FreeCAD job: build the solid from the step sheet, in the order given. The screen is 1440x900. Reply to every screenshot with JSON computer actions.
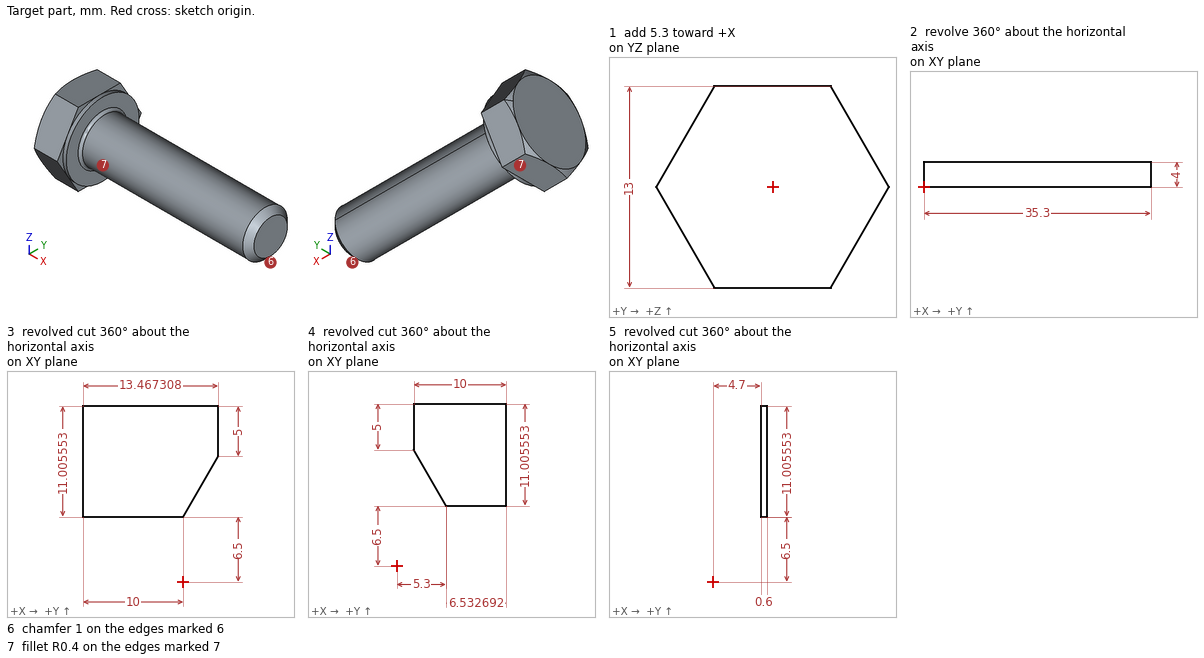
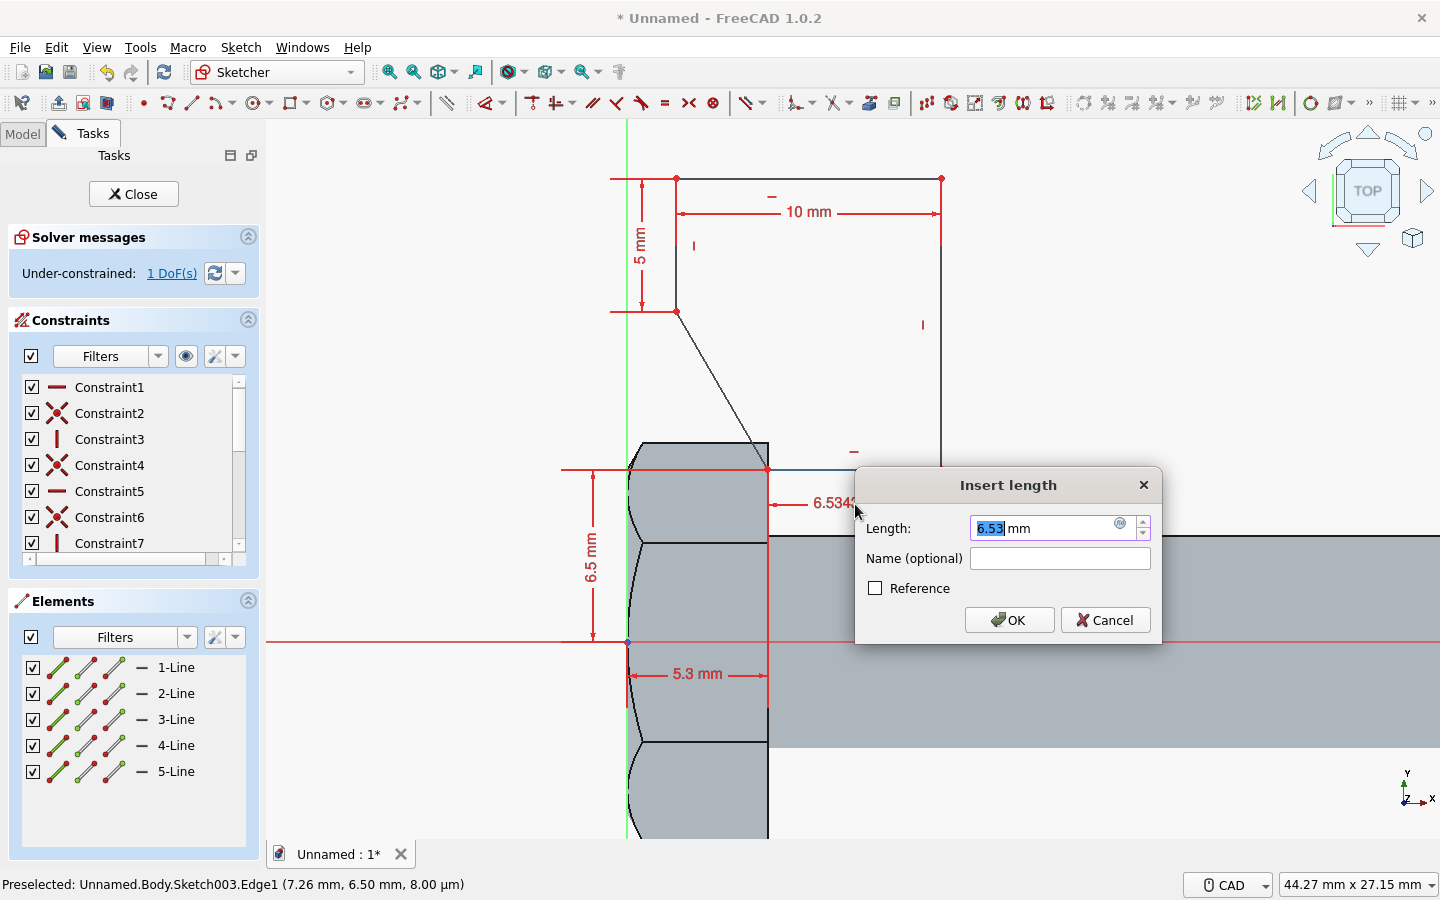
{"action": "type", "text": "6.532692"}
{"action": "key", "text": "Return"}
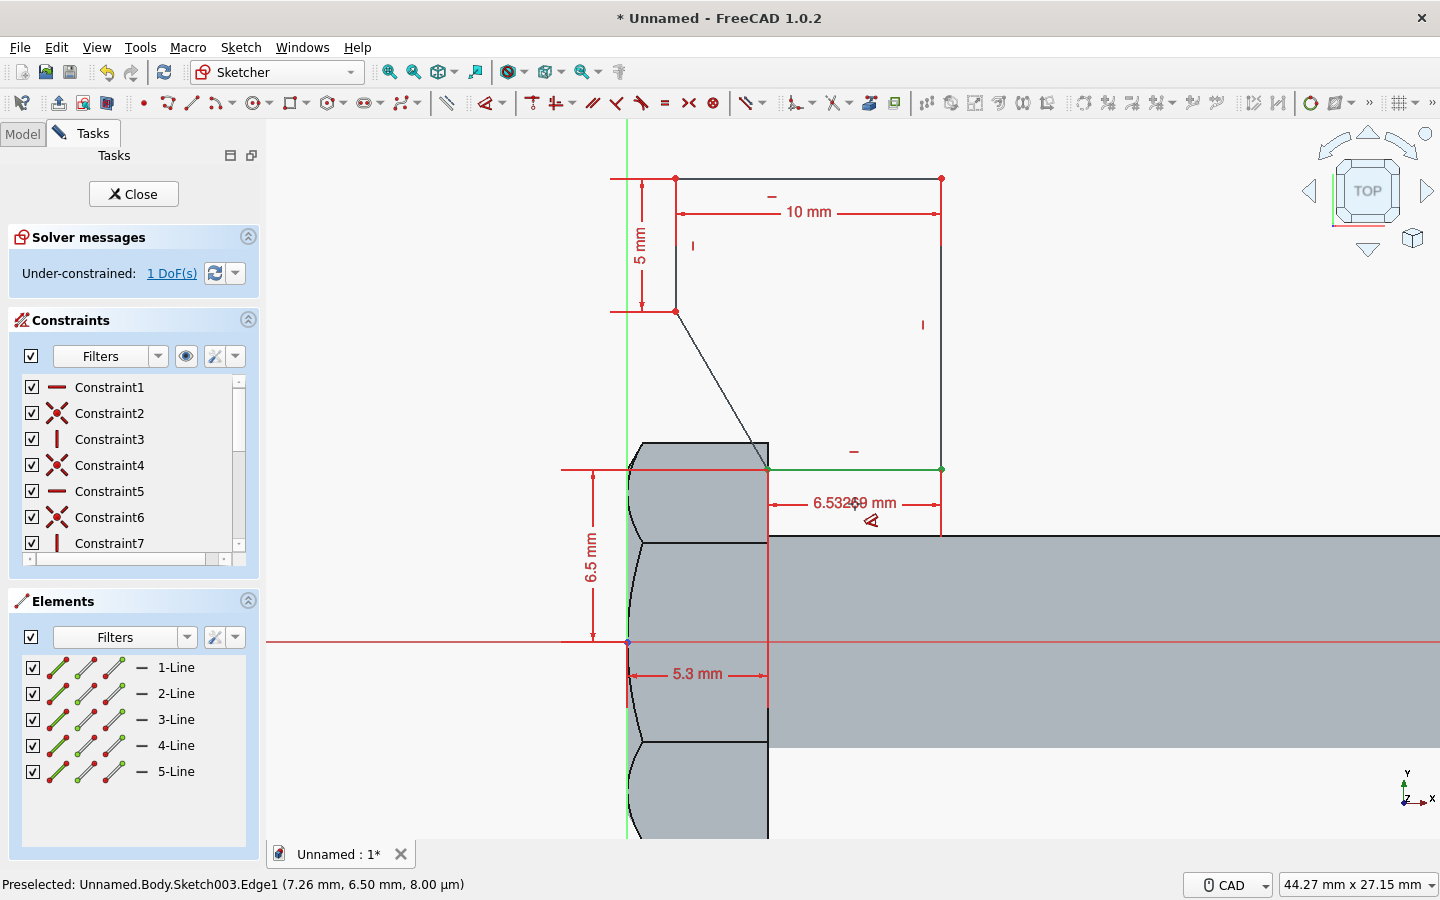
{"action": "left_click", "coordinate": [941, 383]}
{"action": "left_click", "coordinate": [975, 324]}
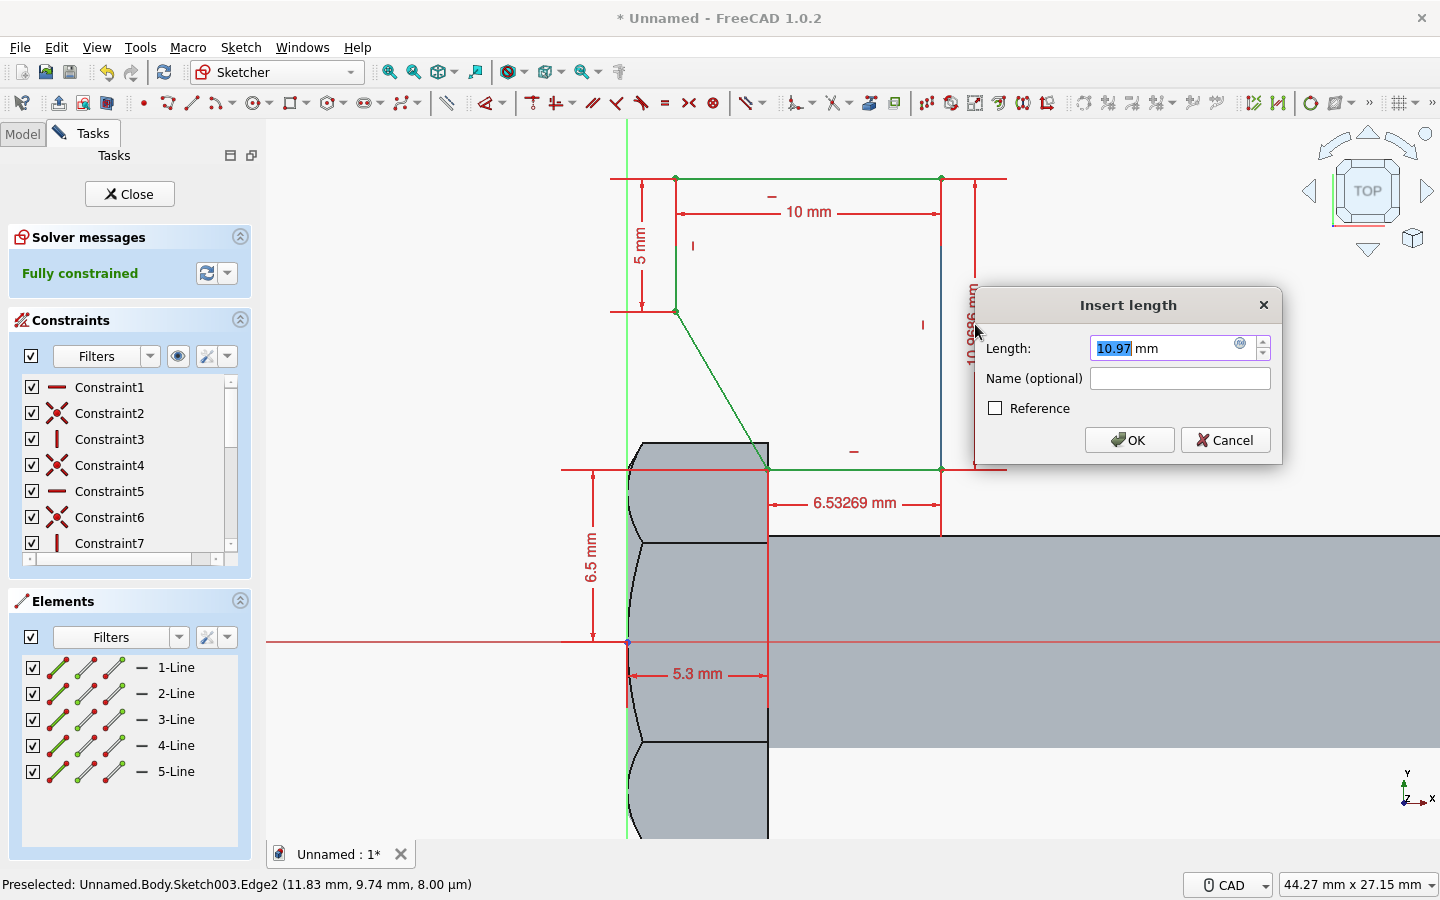
{"action": "type", "text": "11.005553"}
{"action": "key", "text": "Return"}
{"action": "key", "text": "Escape"}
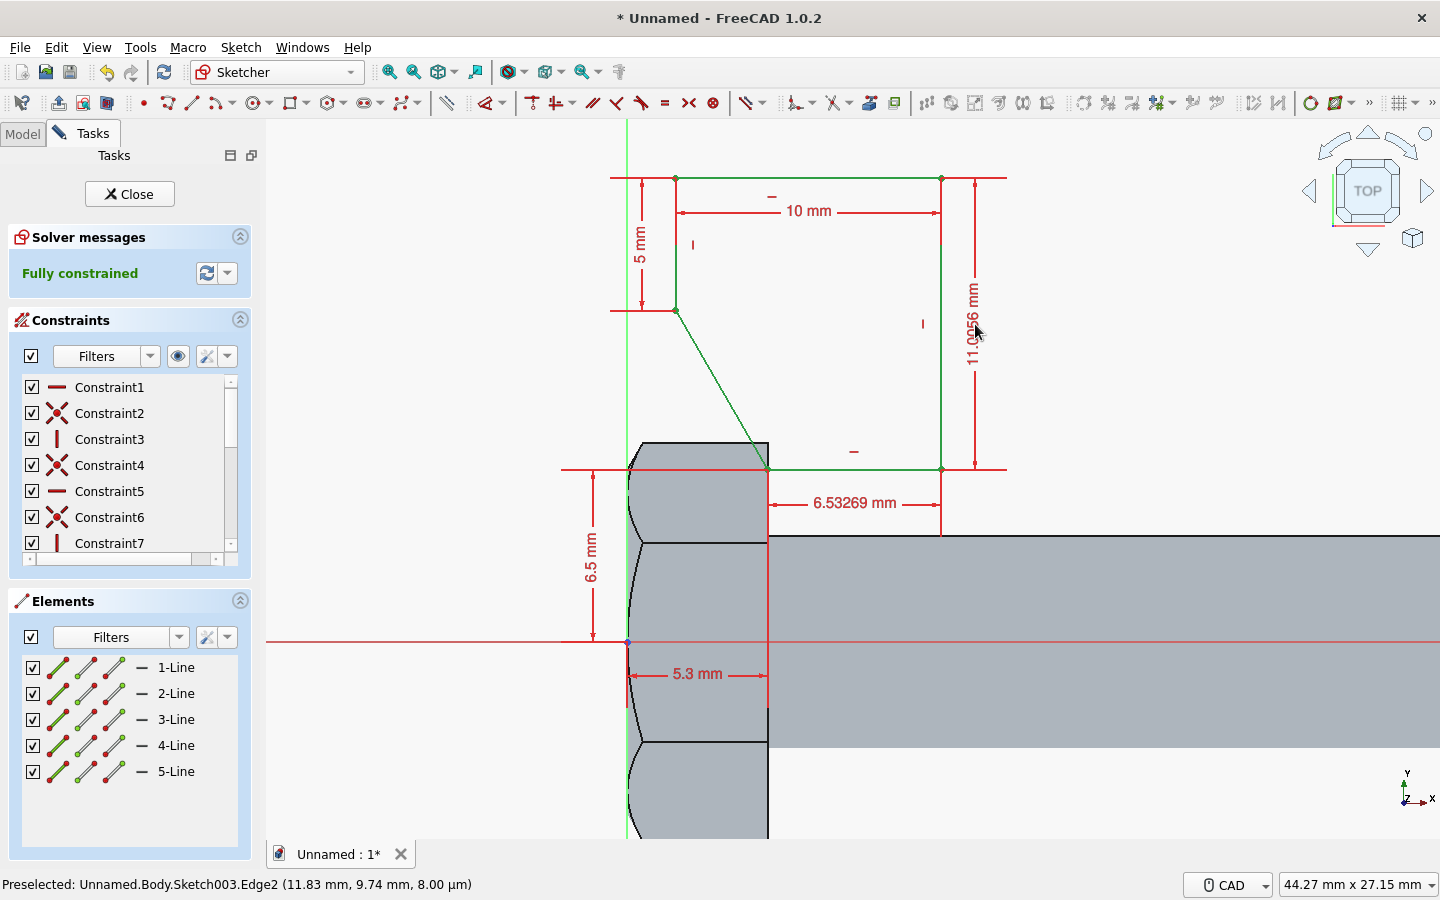
{"action": "left_click", "coordinate": [130, 194]}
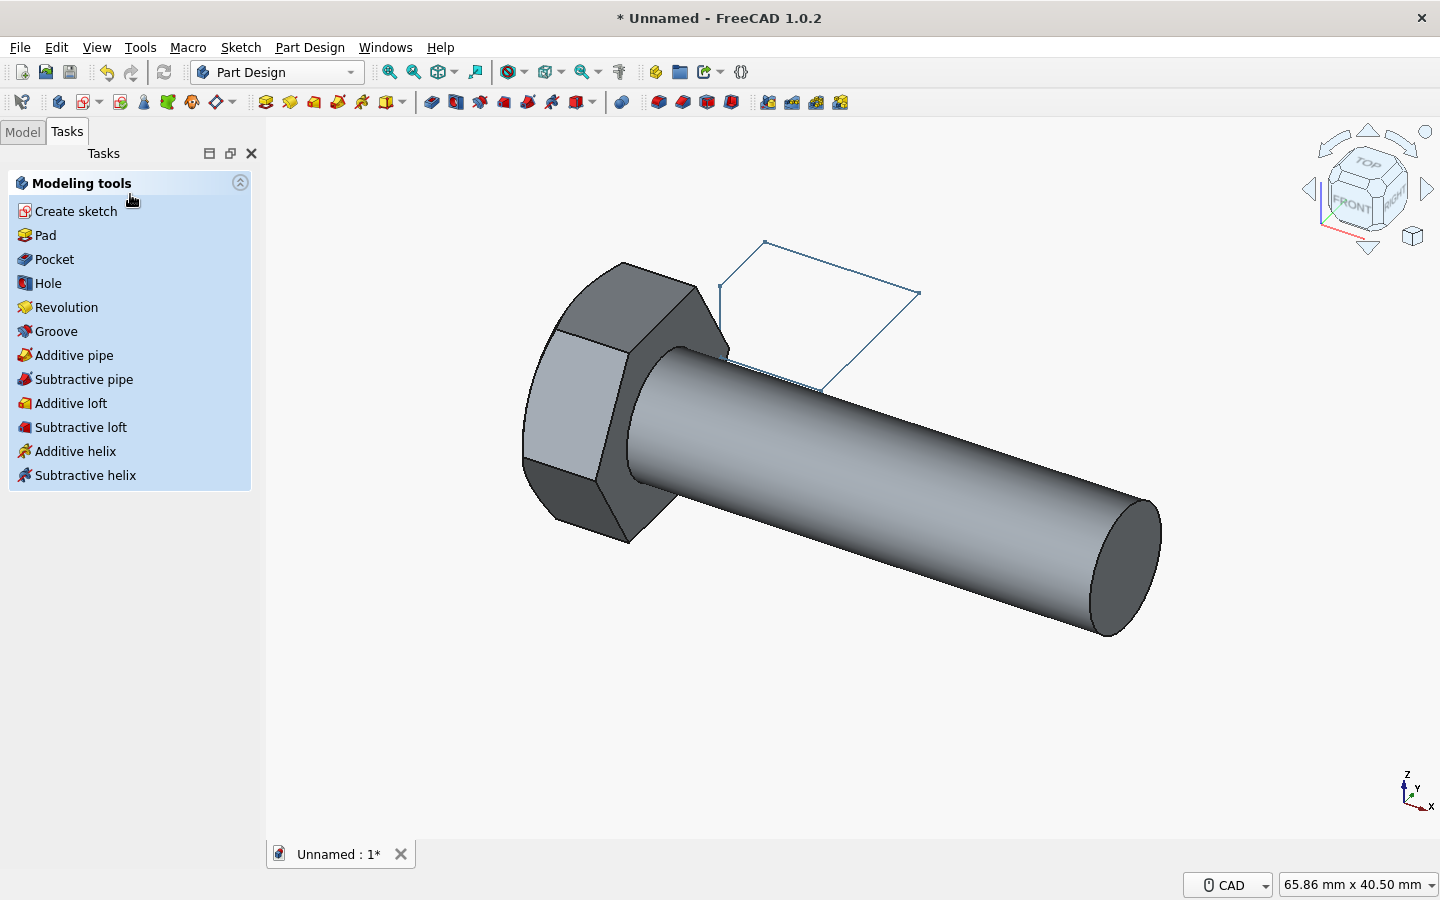
{"action": "left_click", "coordinate": [480, 102]}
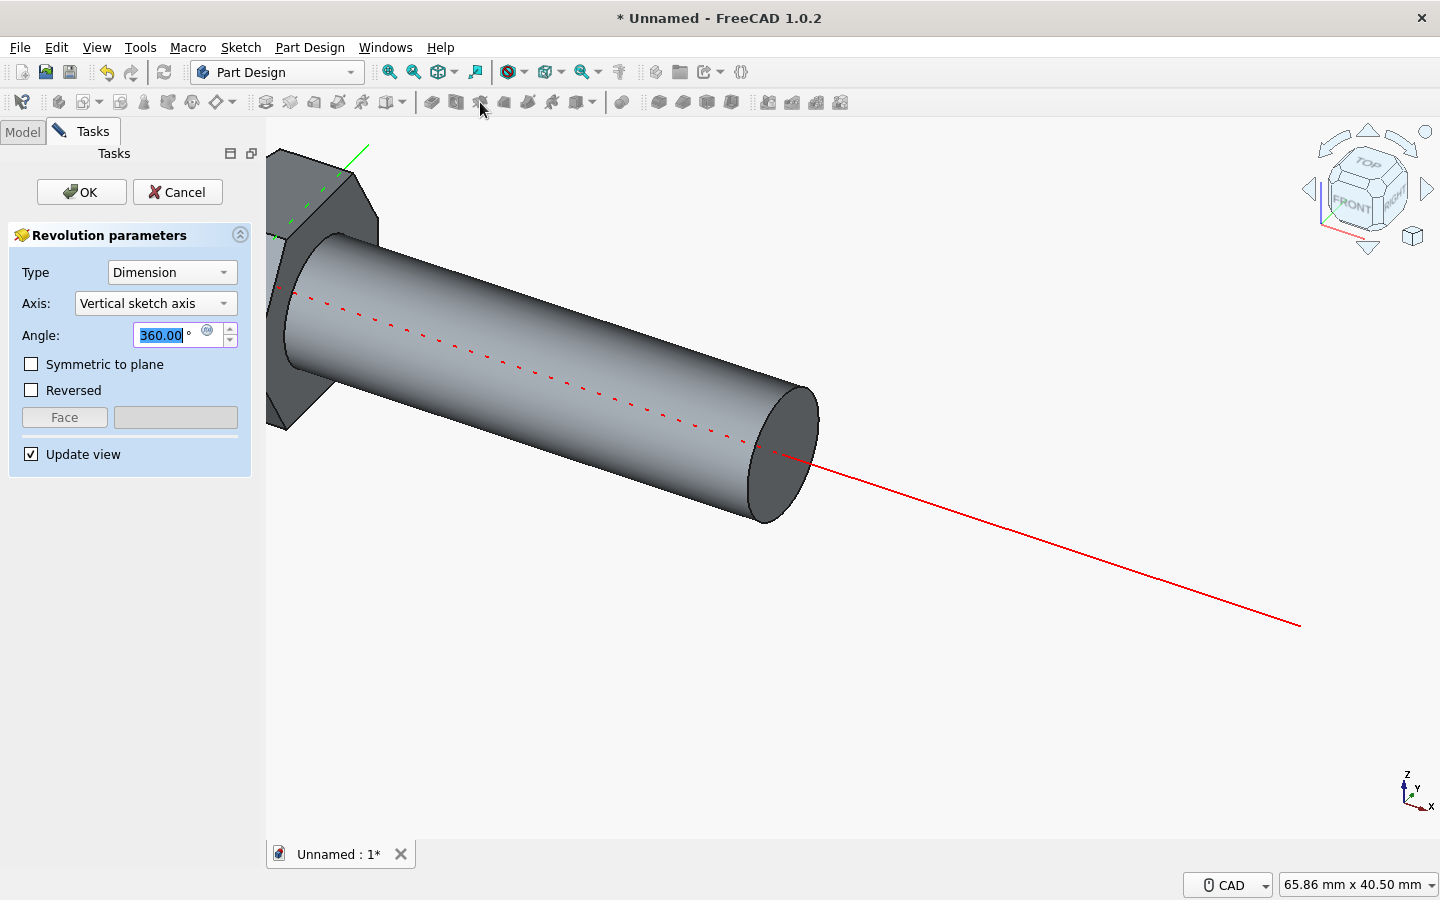
{"action": "left_click", "coordinate": [156, 304]}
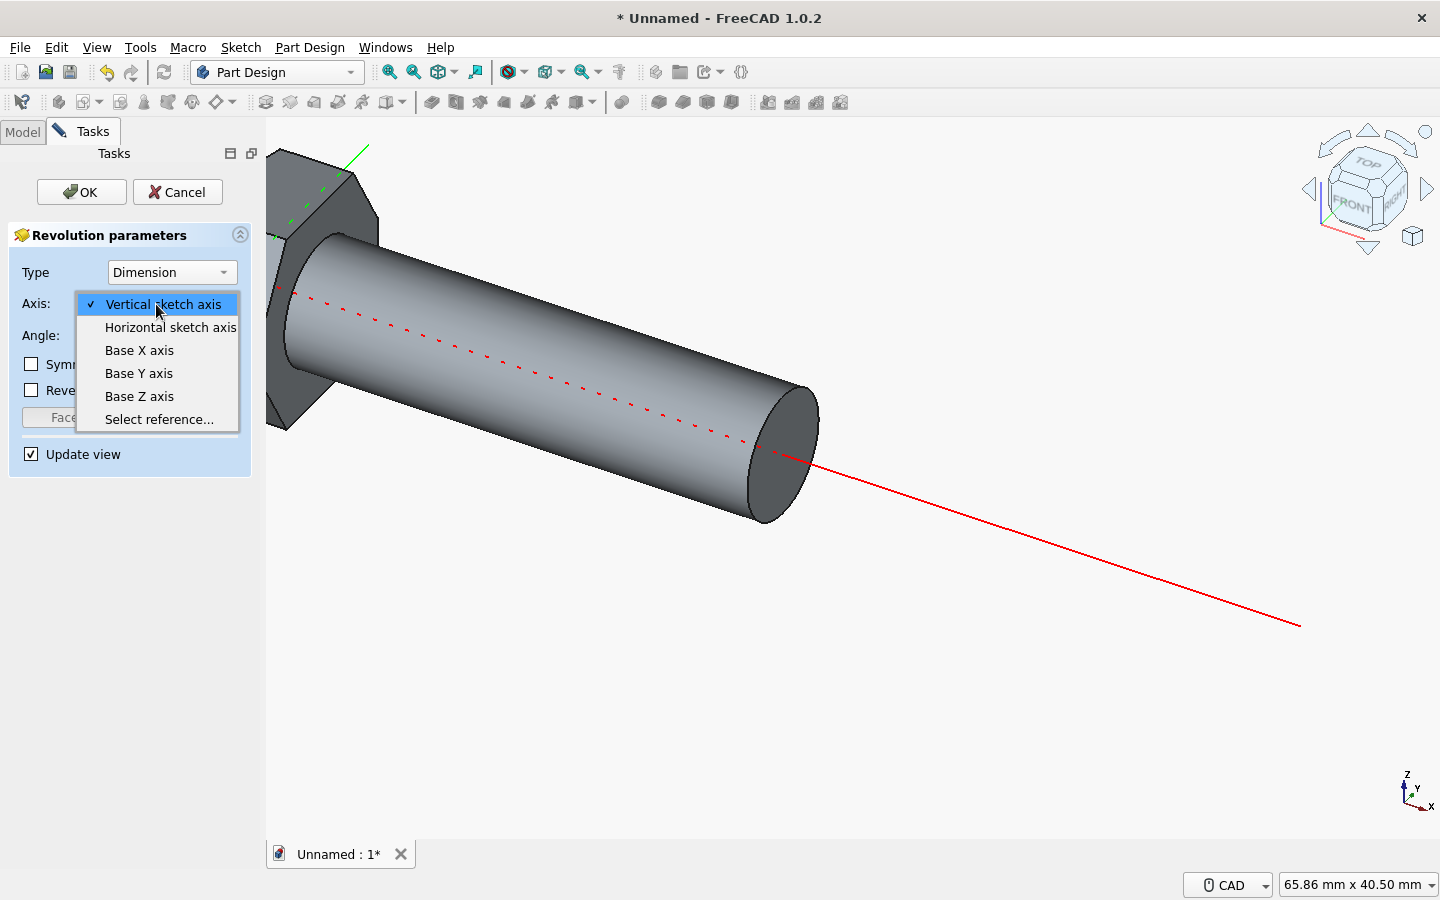
{"action": "left_click", "coordinate": [156, 328]}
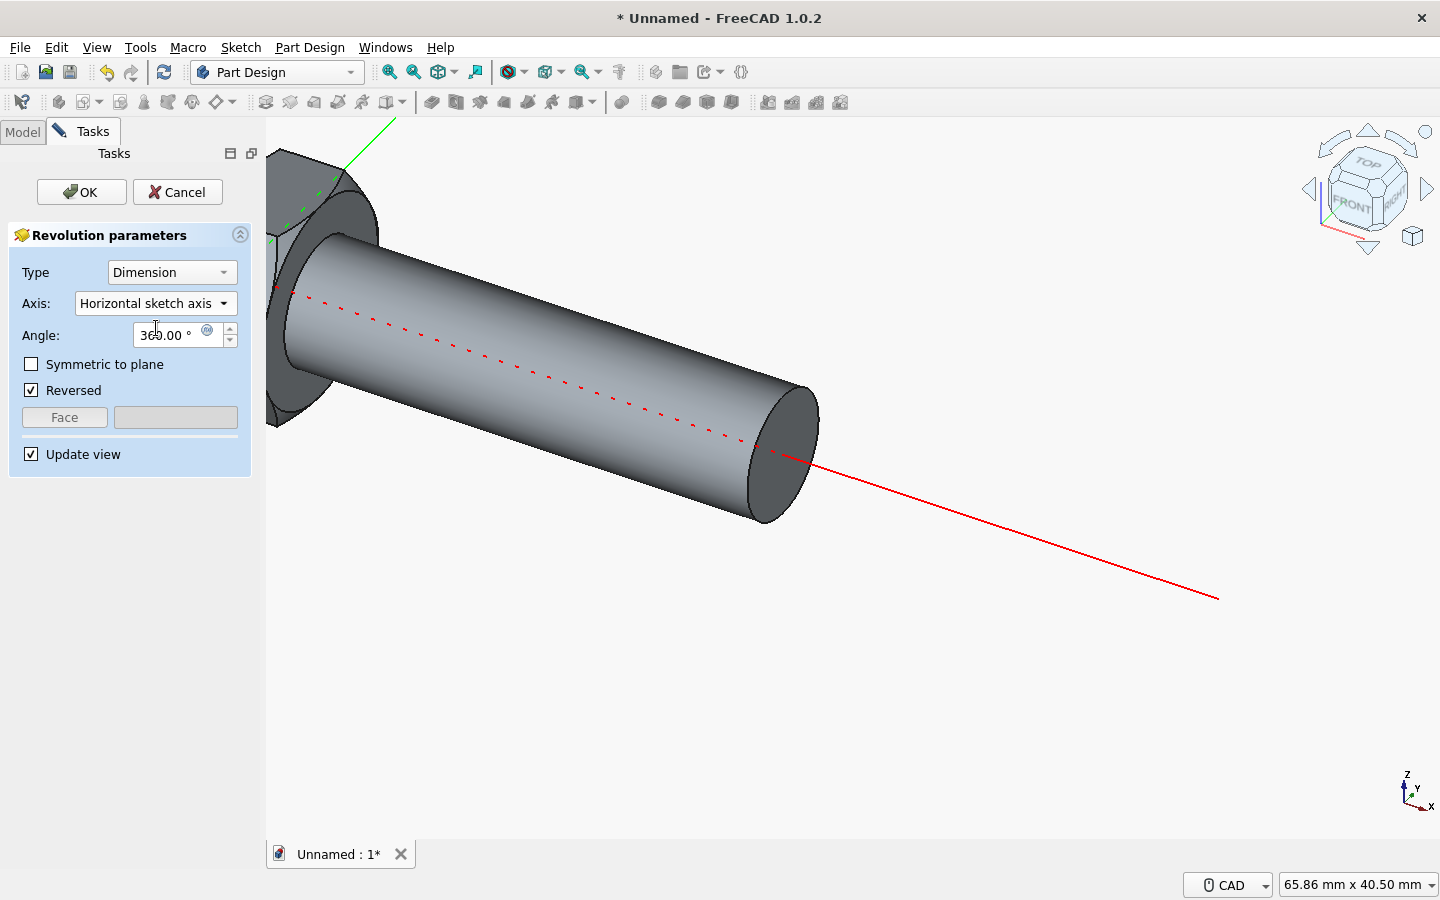
{"action": "left_click", "coordinate": [82, 192]}